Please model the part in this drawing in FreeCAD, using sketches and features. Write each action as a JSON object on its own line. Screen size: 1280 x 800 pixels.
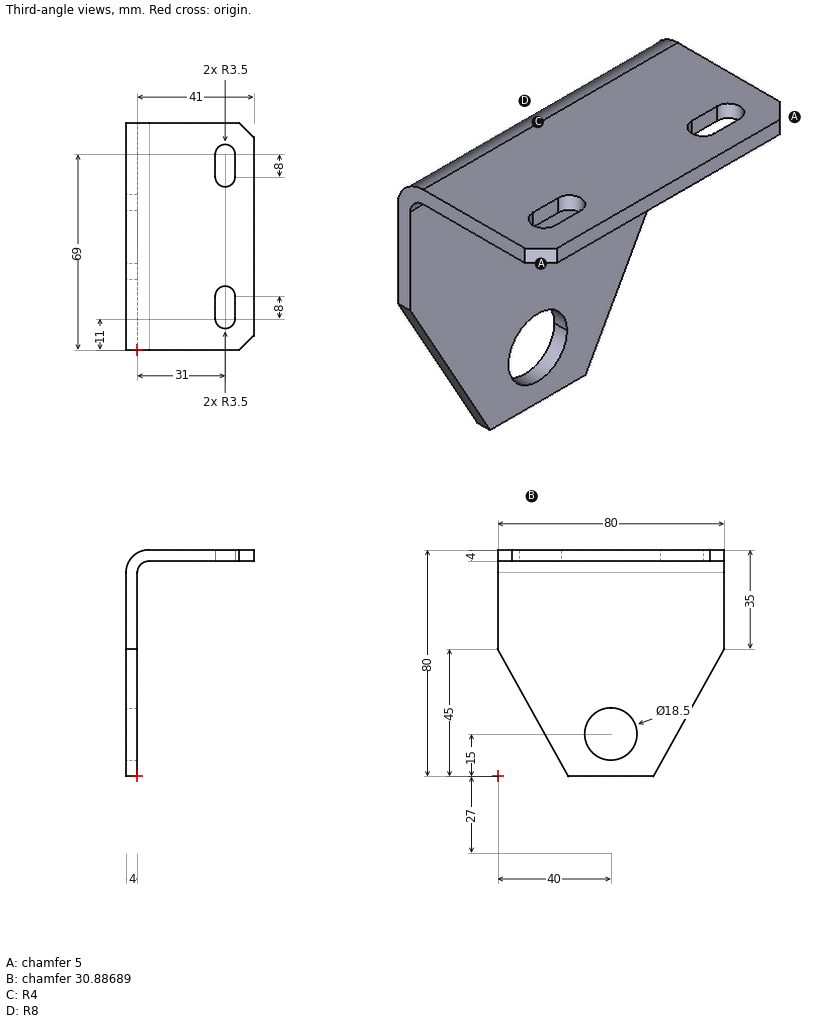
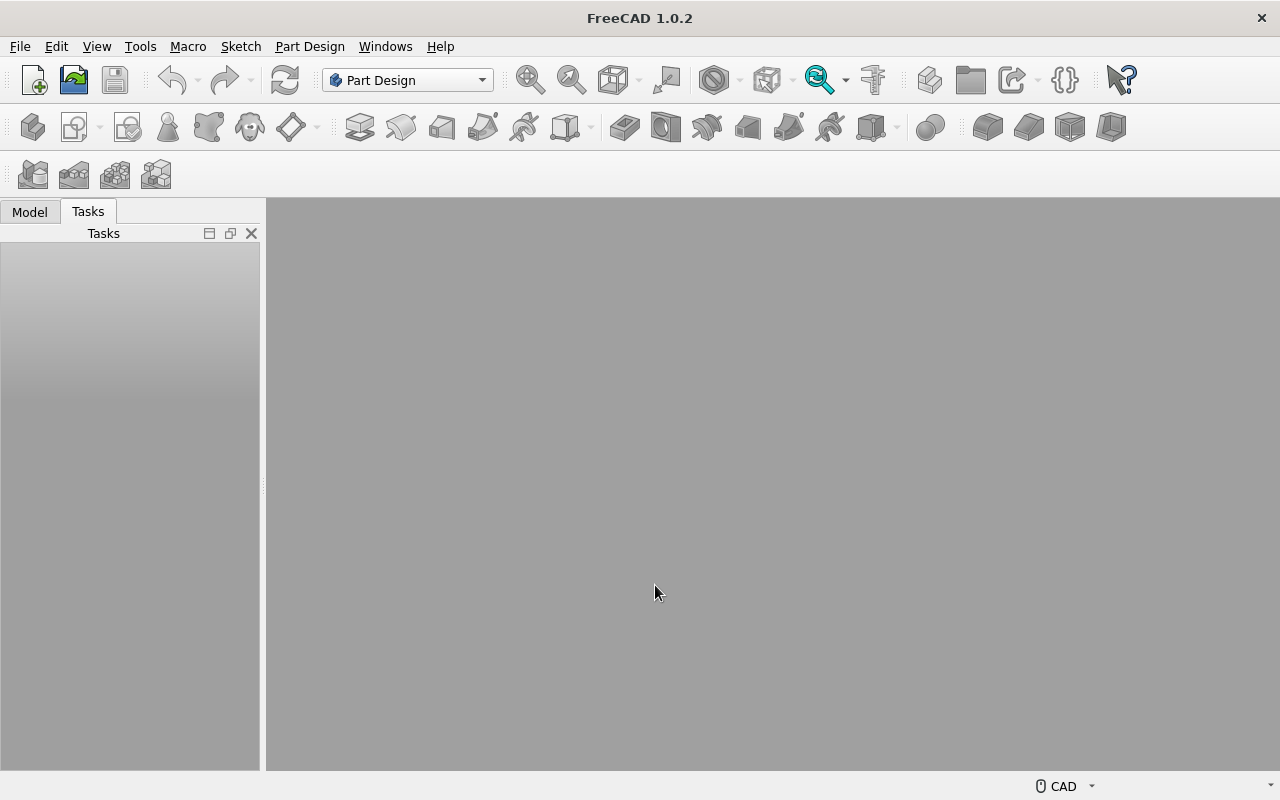
{"action": "key", "text": "ctrl+n"}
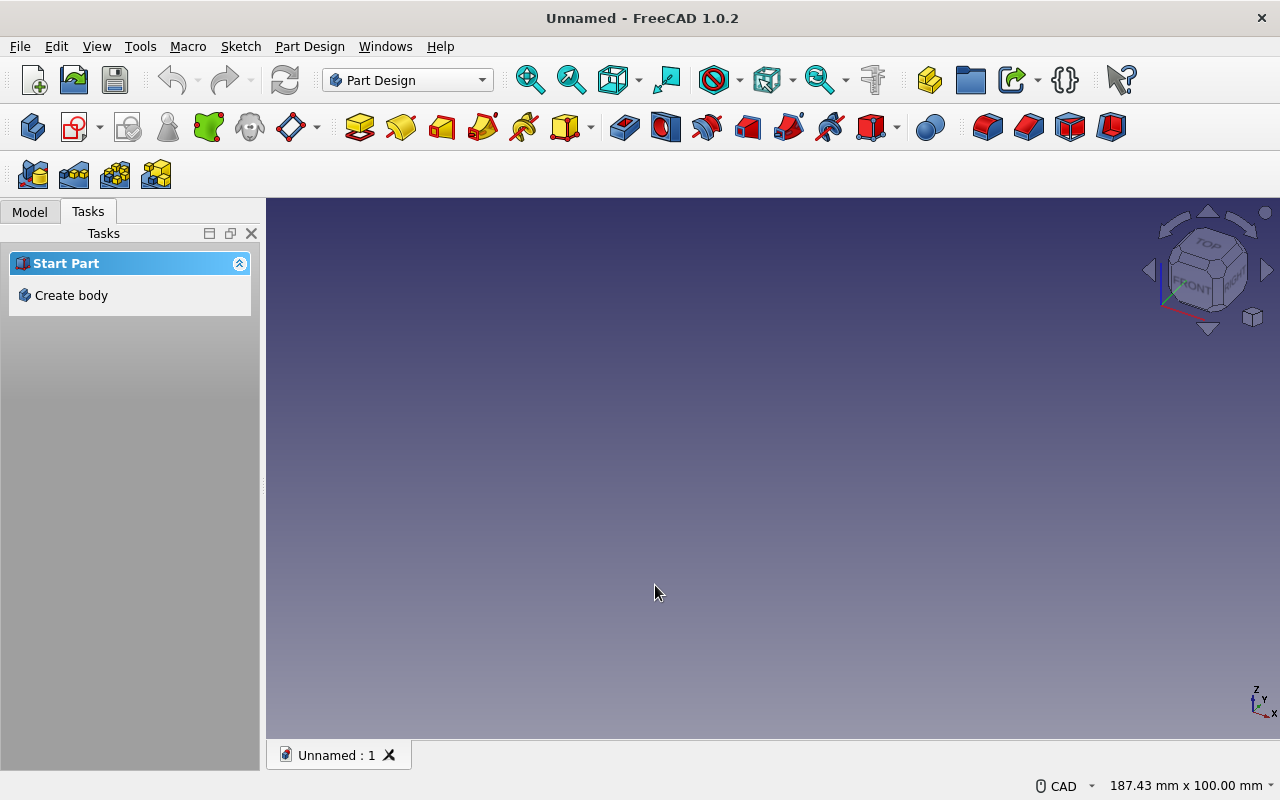
{"action": "left_click", "coordinate": [74, 128]}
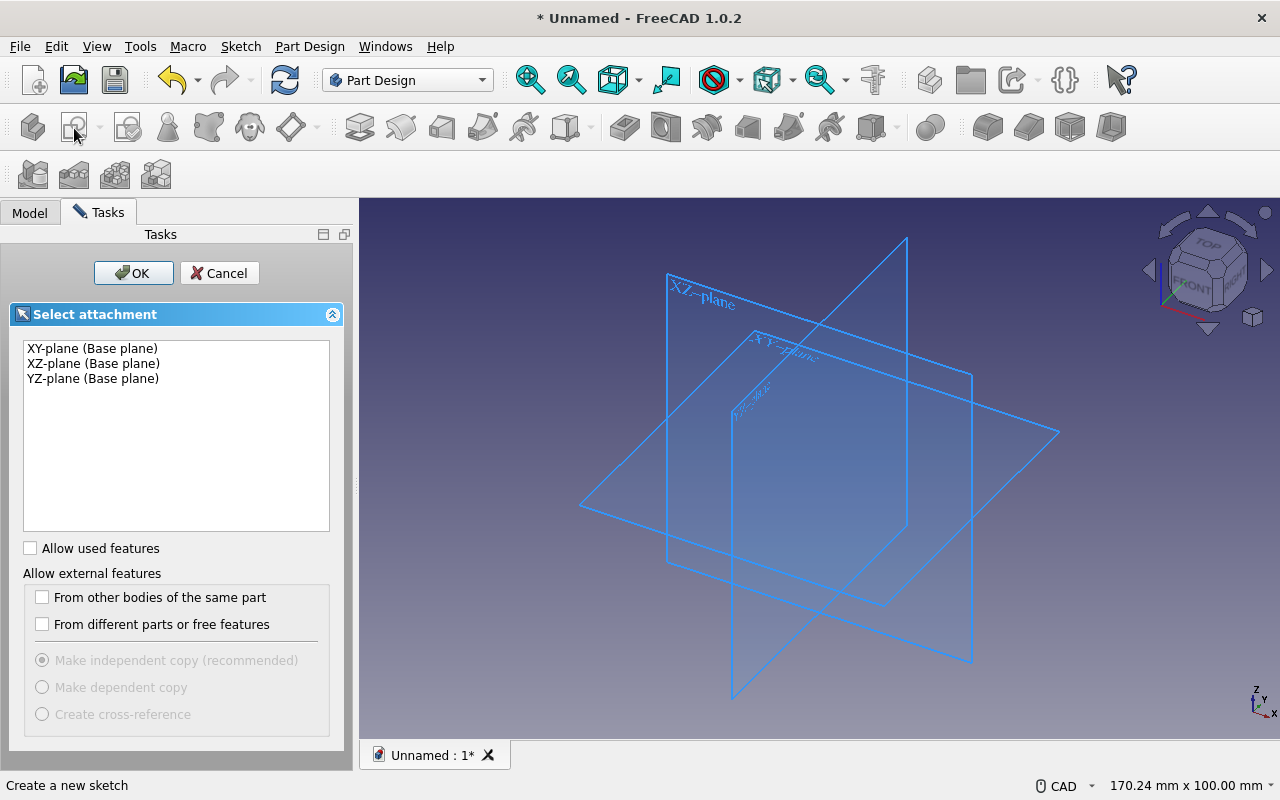
{"action": "left_click", "coordinate": [84, 378]}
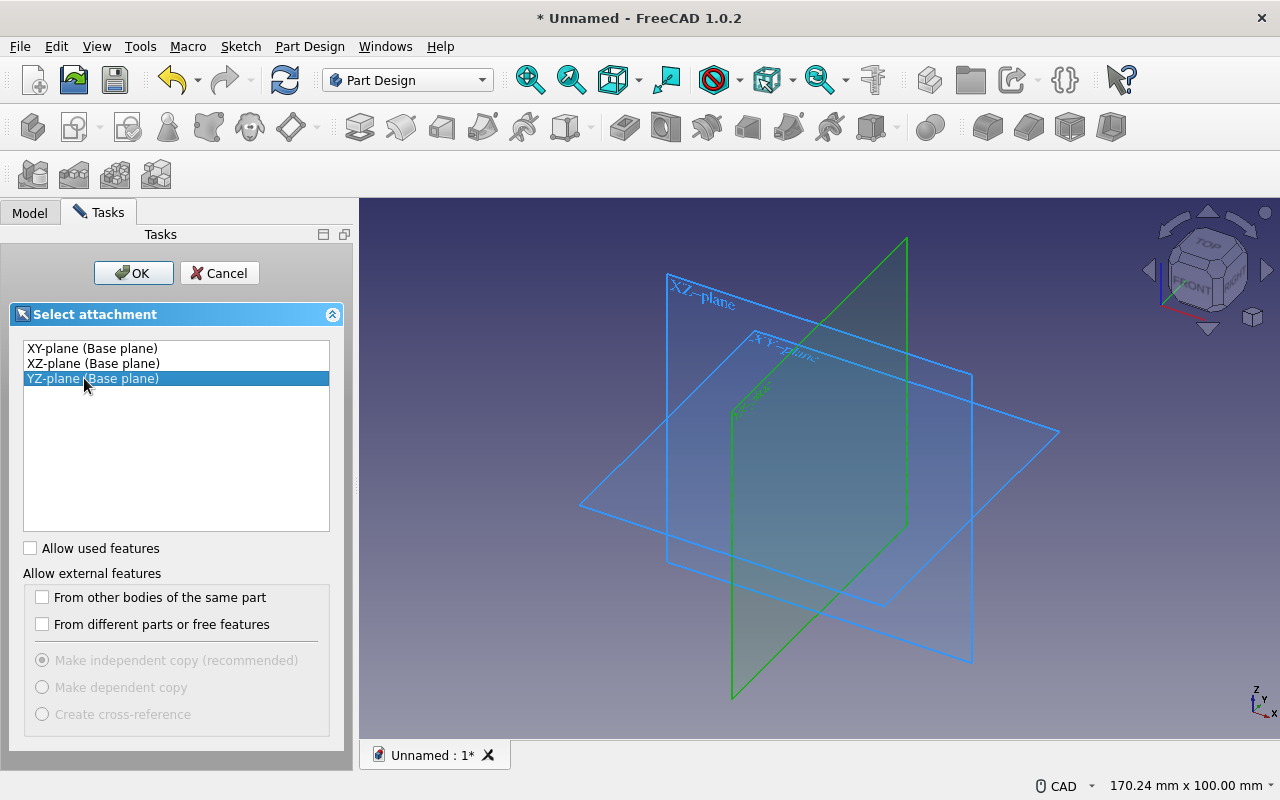
{"action": "left_click", "coordinate": [134, 273]}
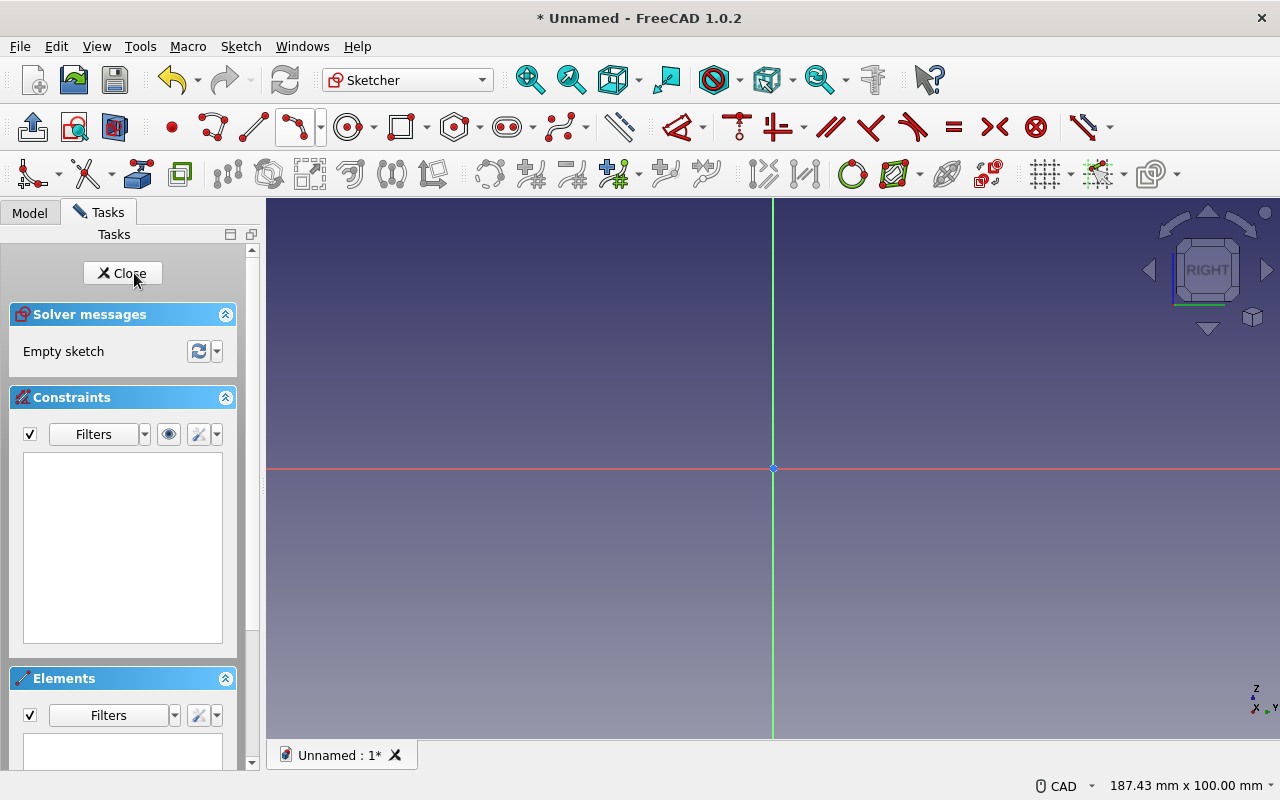
{"action": "scroll", "coordinate": [358, 643], "scroll_direction": "down", "scroll_amount": 3}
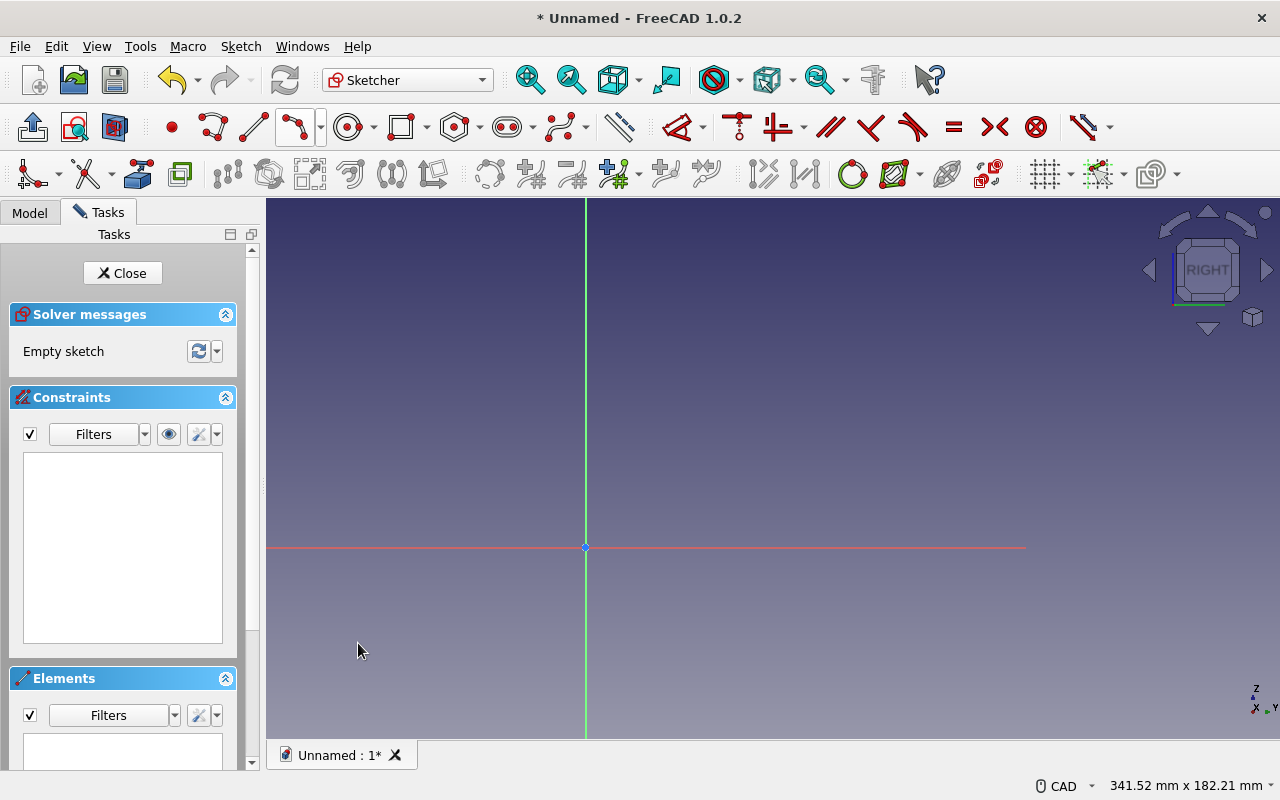
{"action": "key", "text": "g m"}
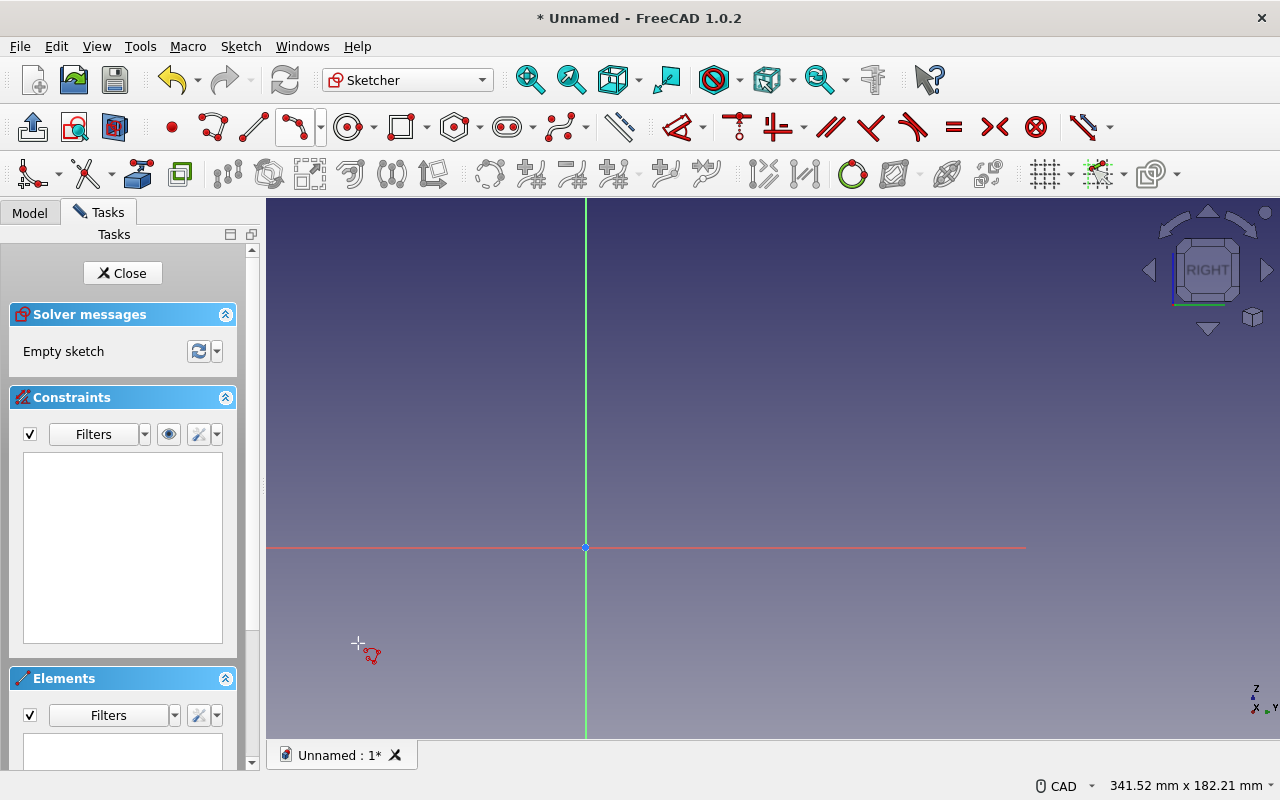
{"action": "left_click", "coordinate": [586, 414]}
{"action": "left_click", "coordinate": [705, 628]}
{"action": "left_click", "coordinate": [823, 414]}
{"action": "left_click", "coordinate": [823, 310]}
{"action": "left_click", "coordinate": [595, 310]}
{"action": "left_click", "coordinate": [586, 415]}
{"action": "key", "text": "Escape"}
{"action": "key", "text": "Escape"}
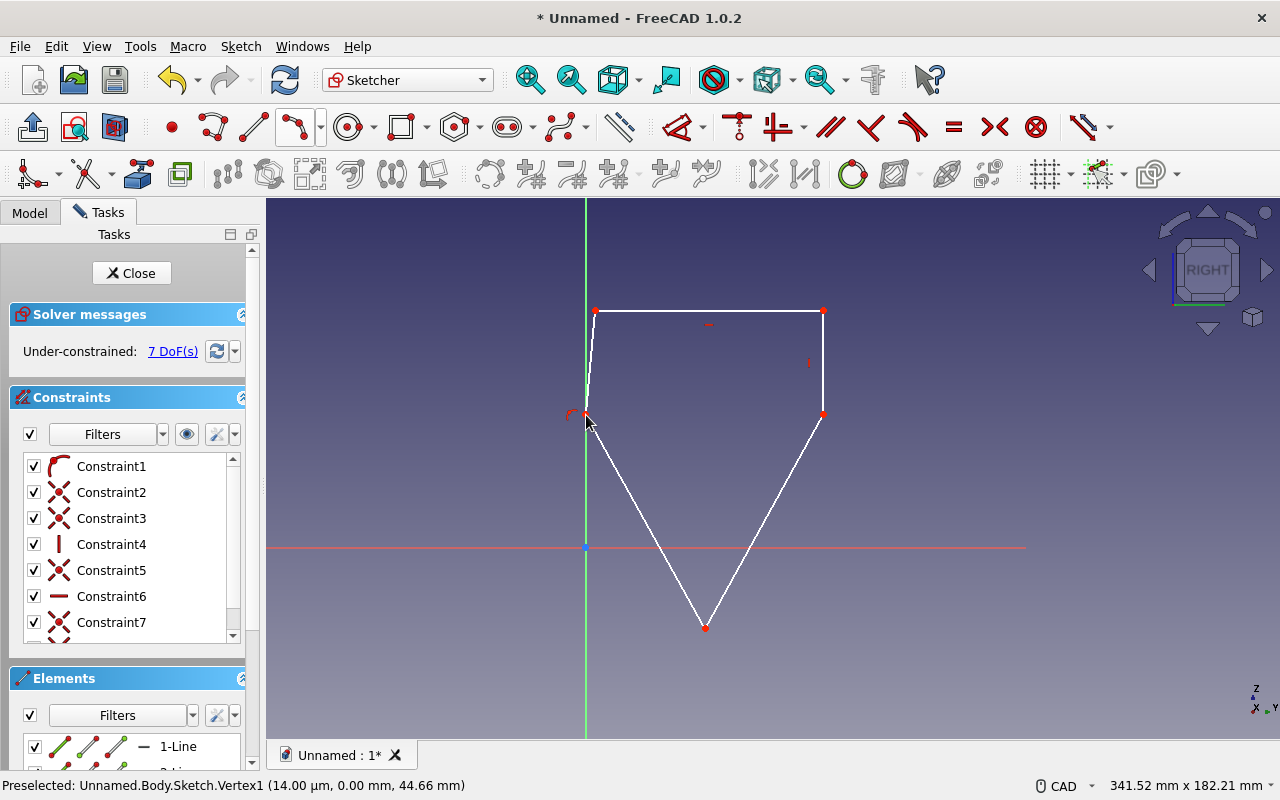
{"action": "left_click", "coordinate": [589, 384]}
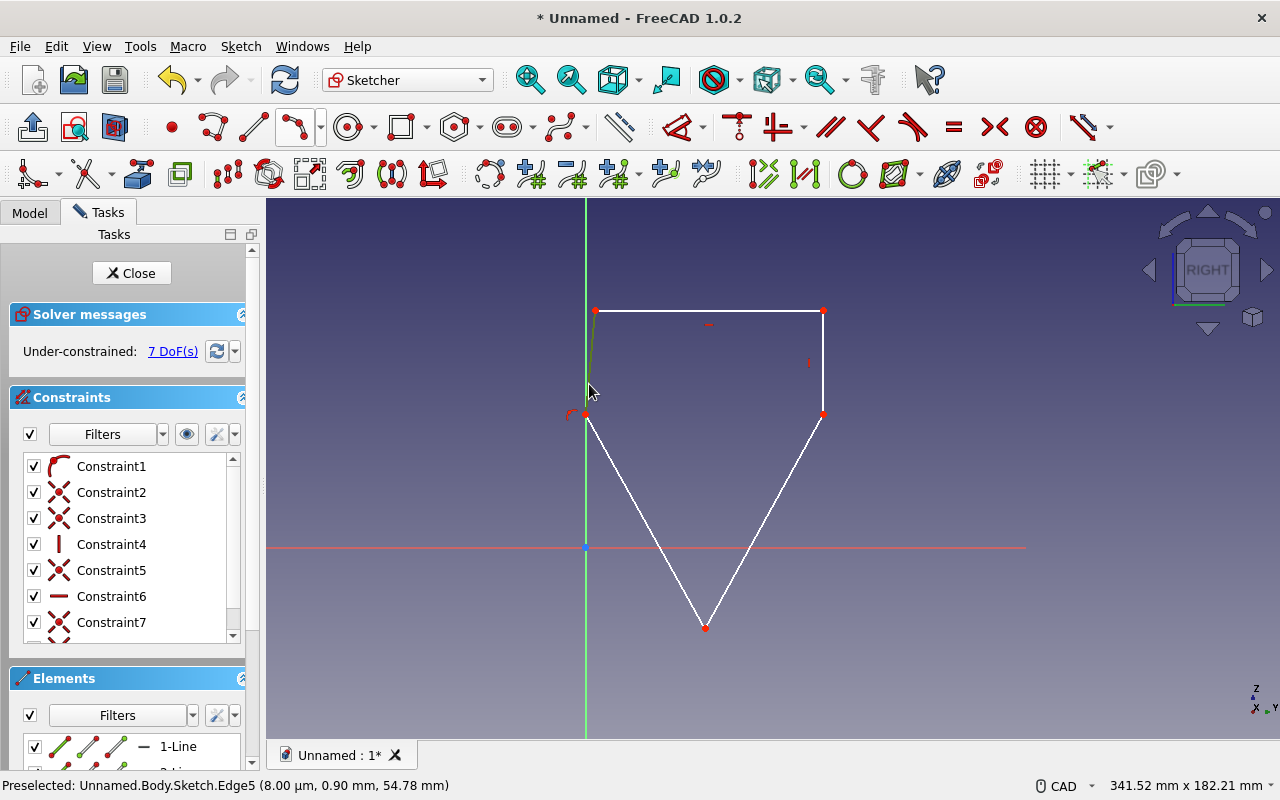
{"action": "key", "text": "v"}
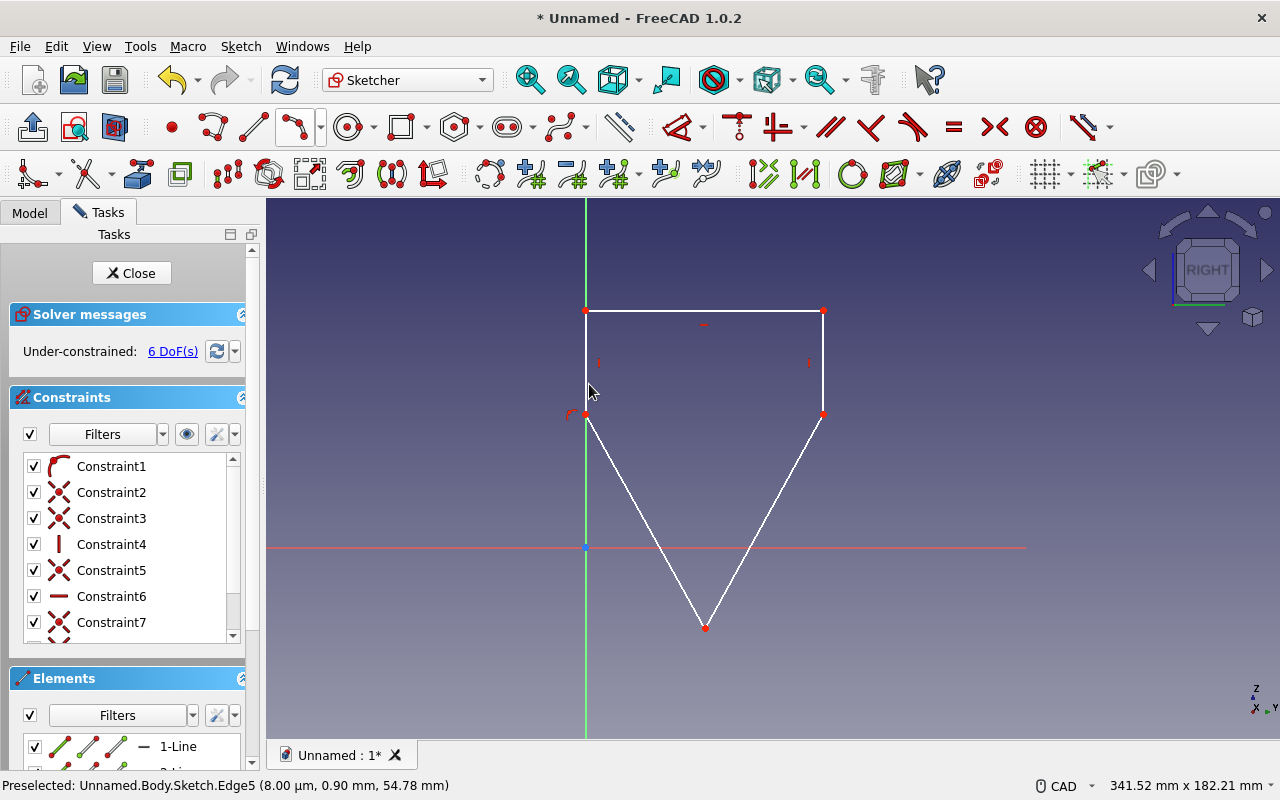
{"action": "key", "text": "d"}